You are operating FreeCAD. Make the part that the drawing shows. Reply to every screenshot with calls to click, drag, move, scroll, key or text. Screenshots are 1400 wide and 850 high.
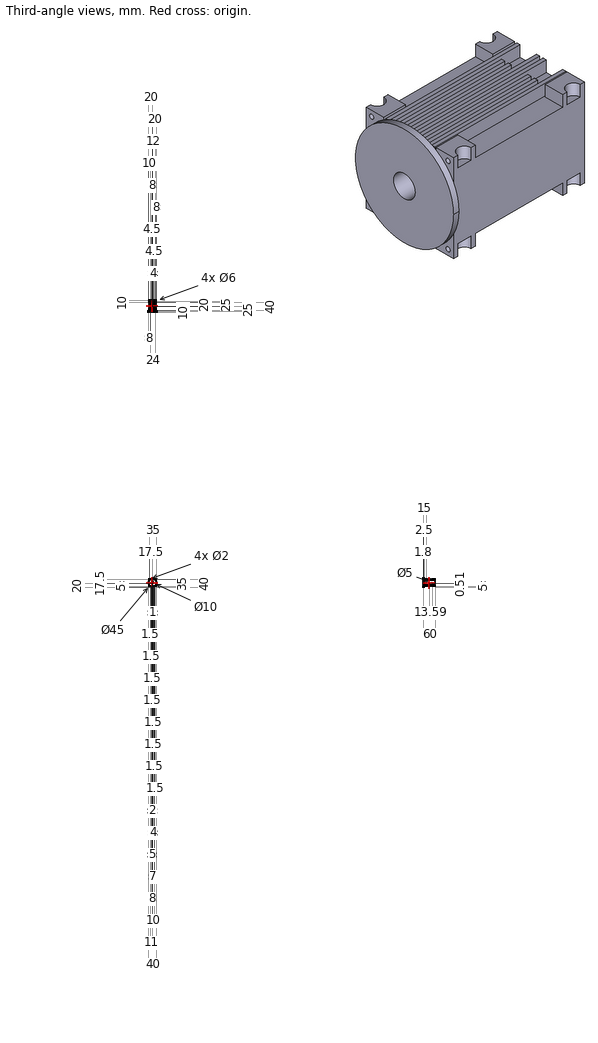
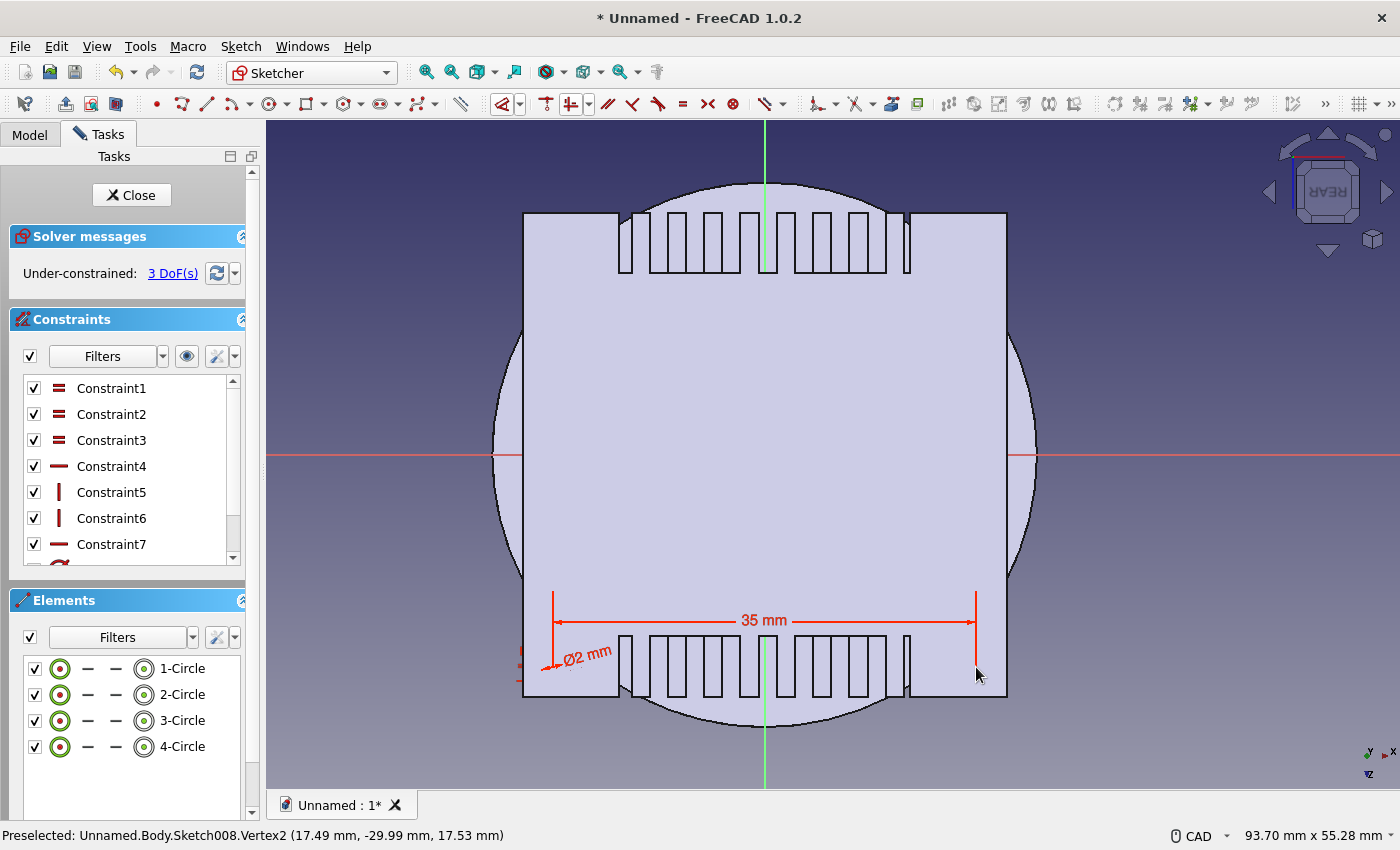
click(976, 667)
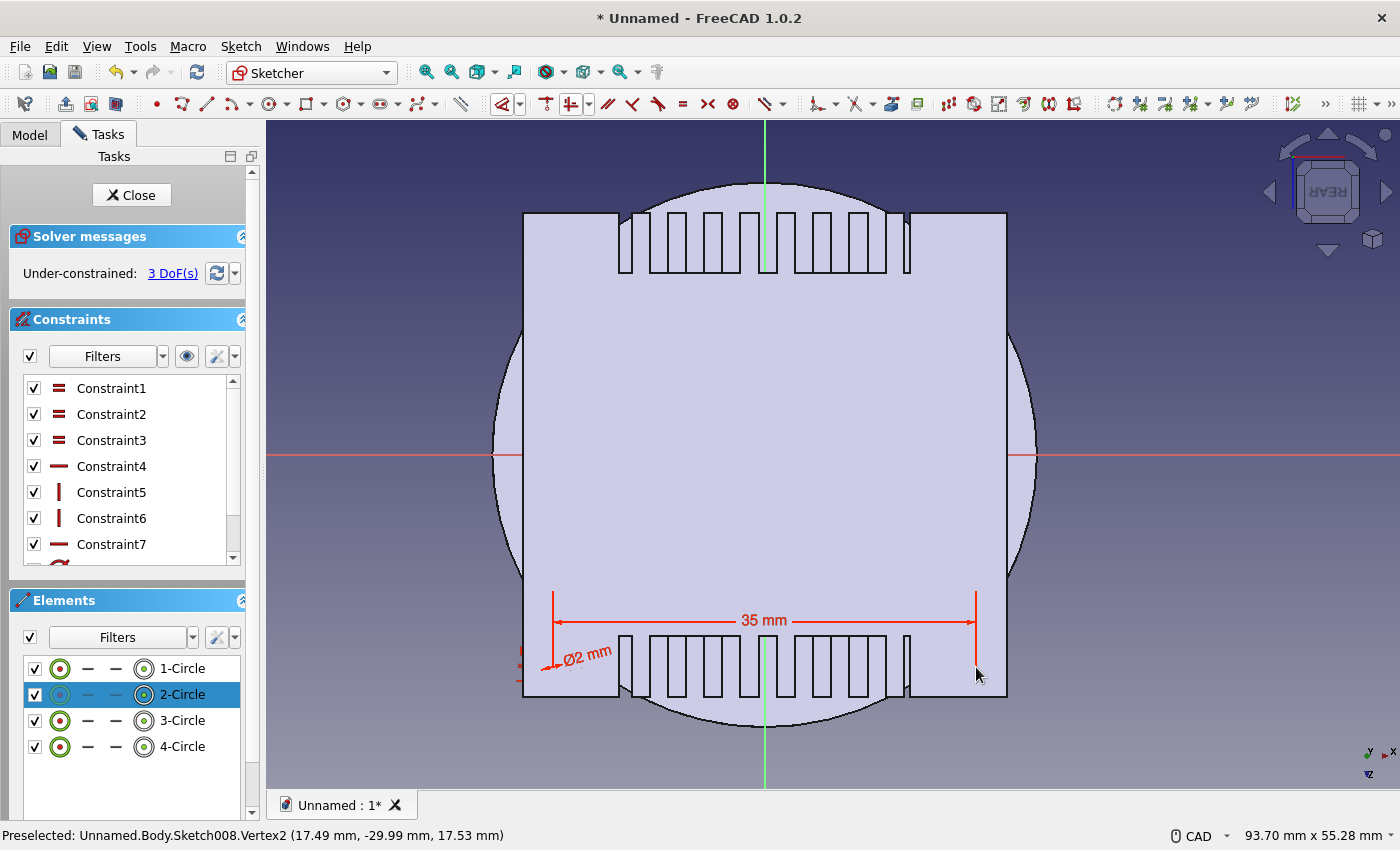
click(976, 244)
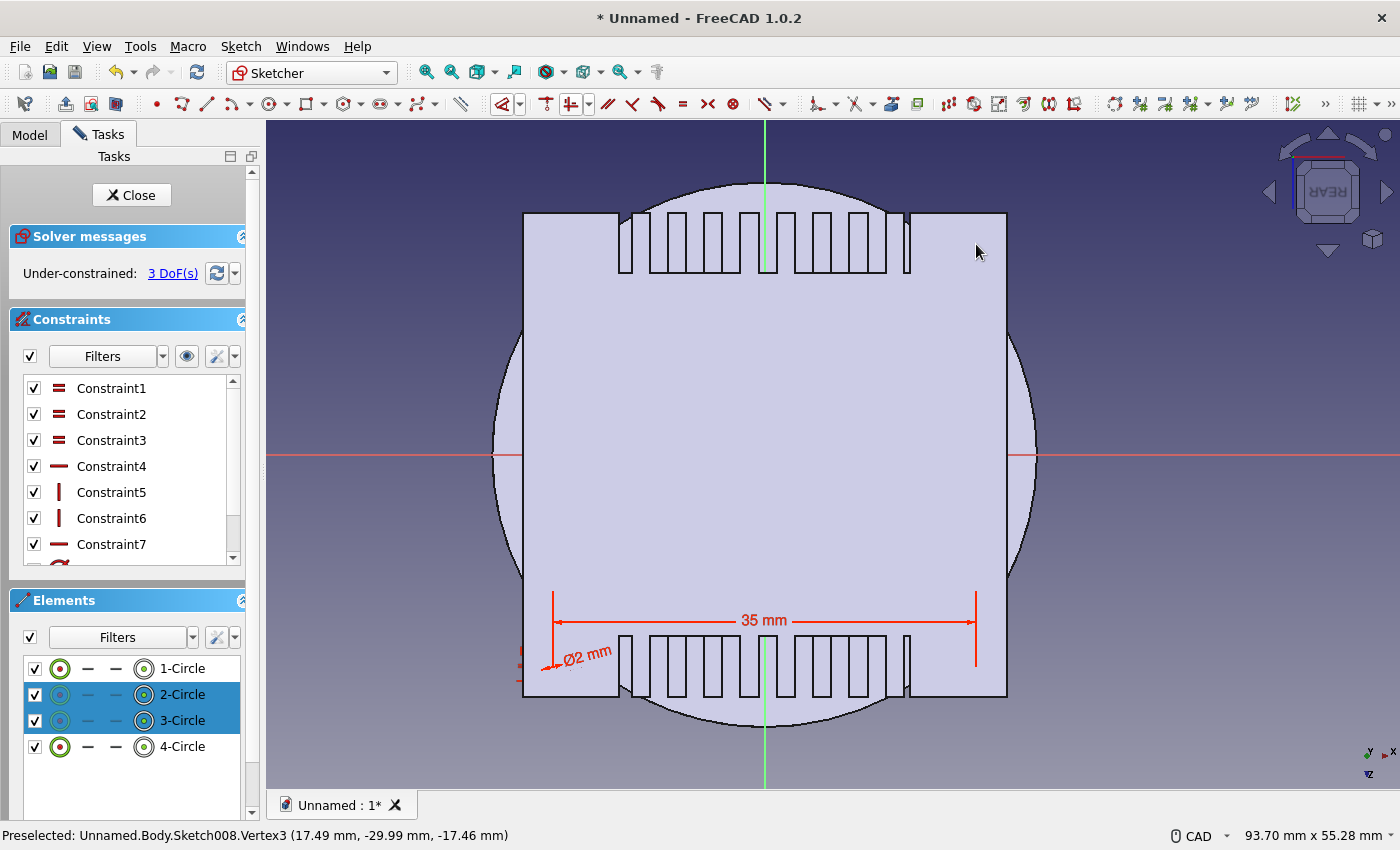
key(i)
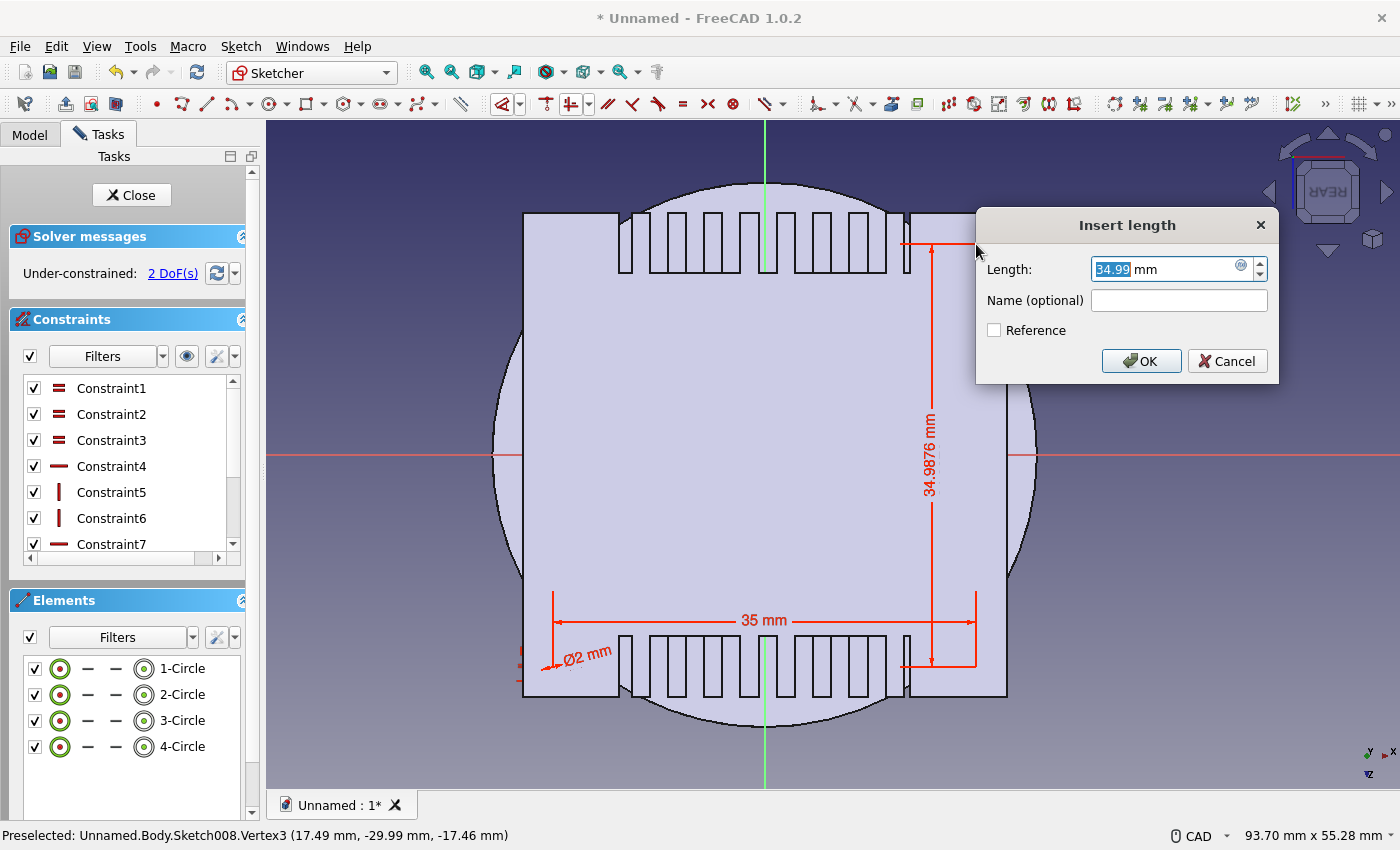
text(35)
key(Return)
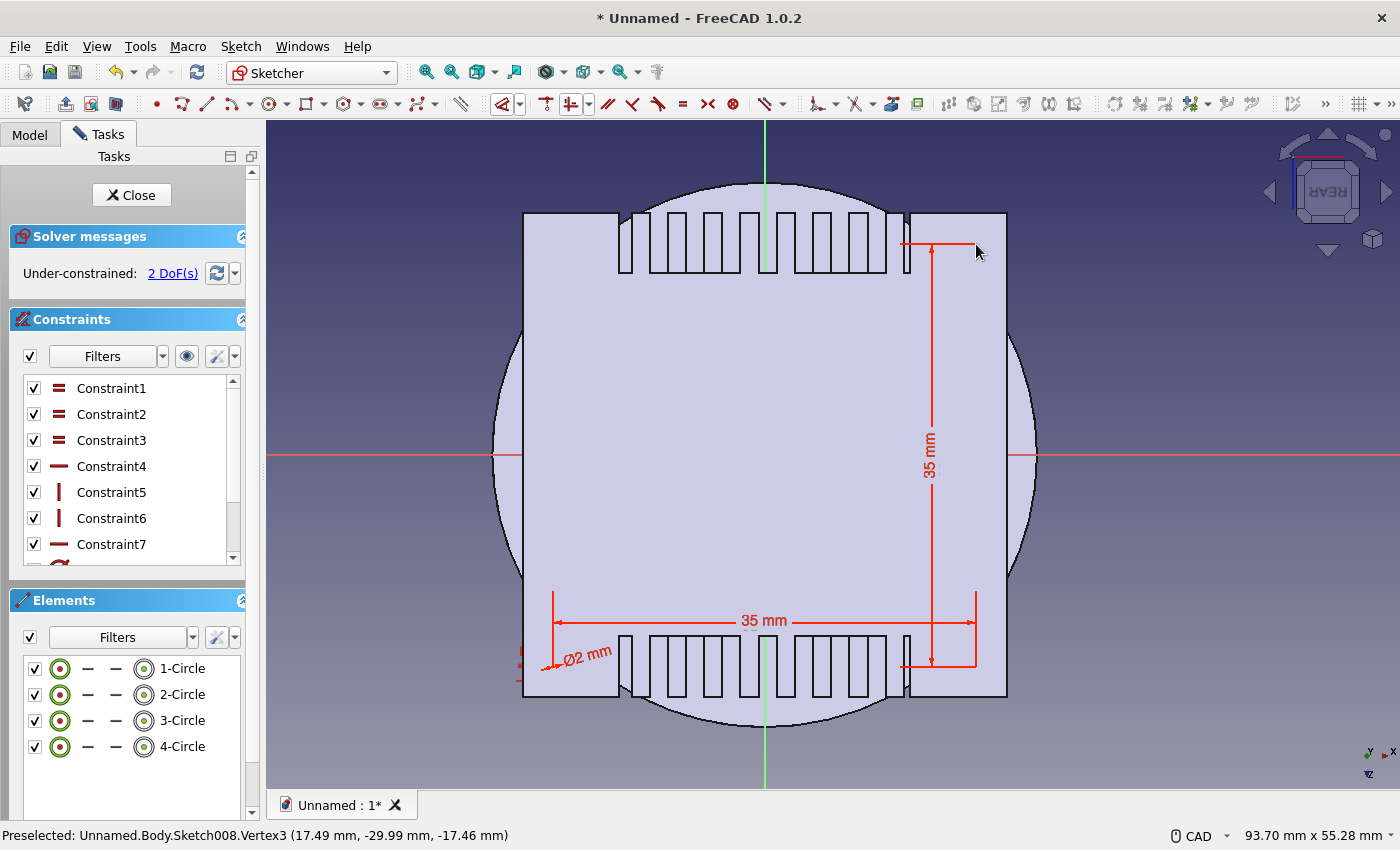
click(553, 667)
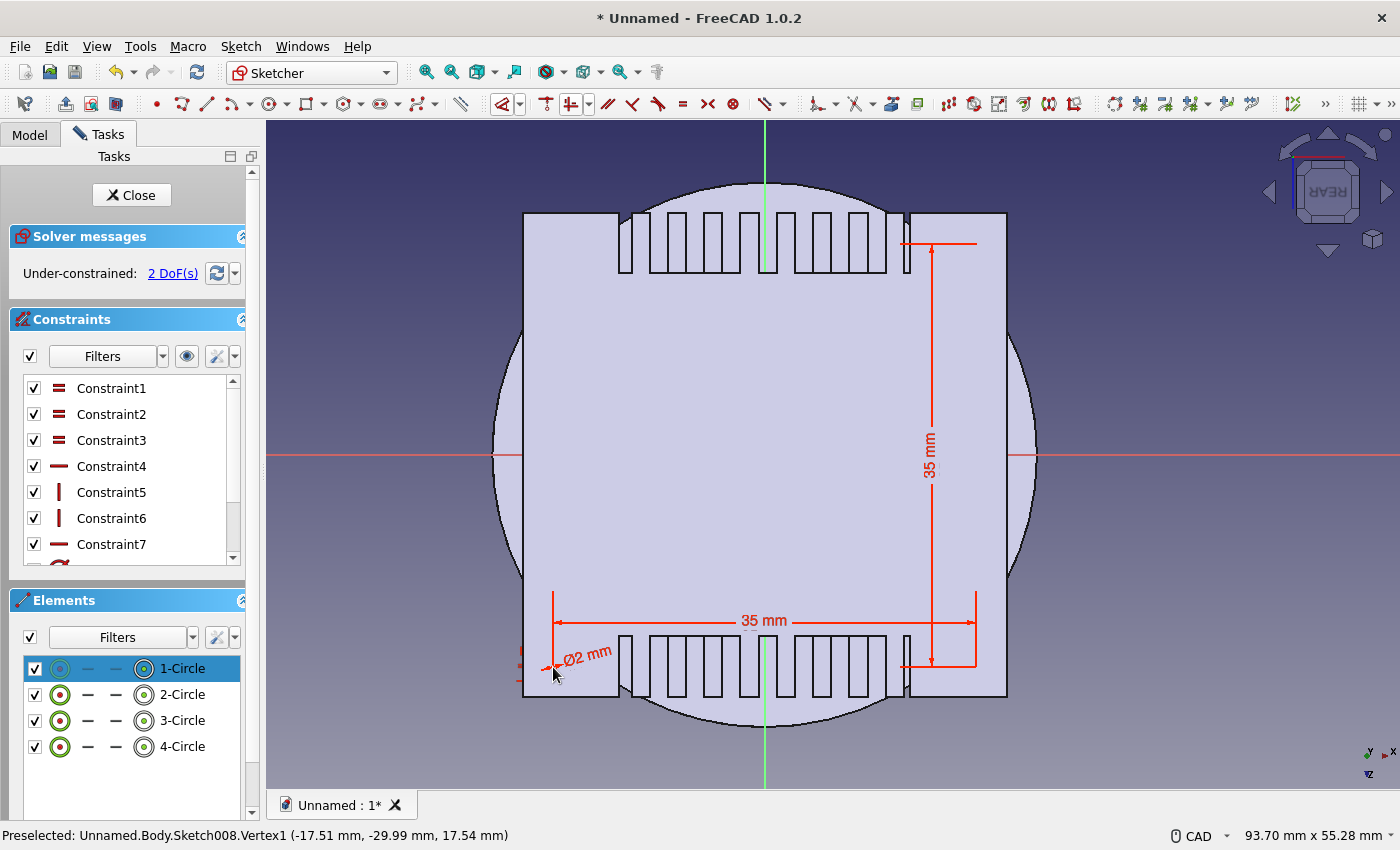
click(520, 104)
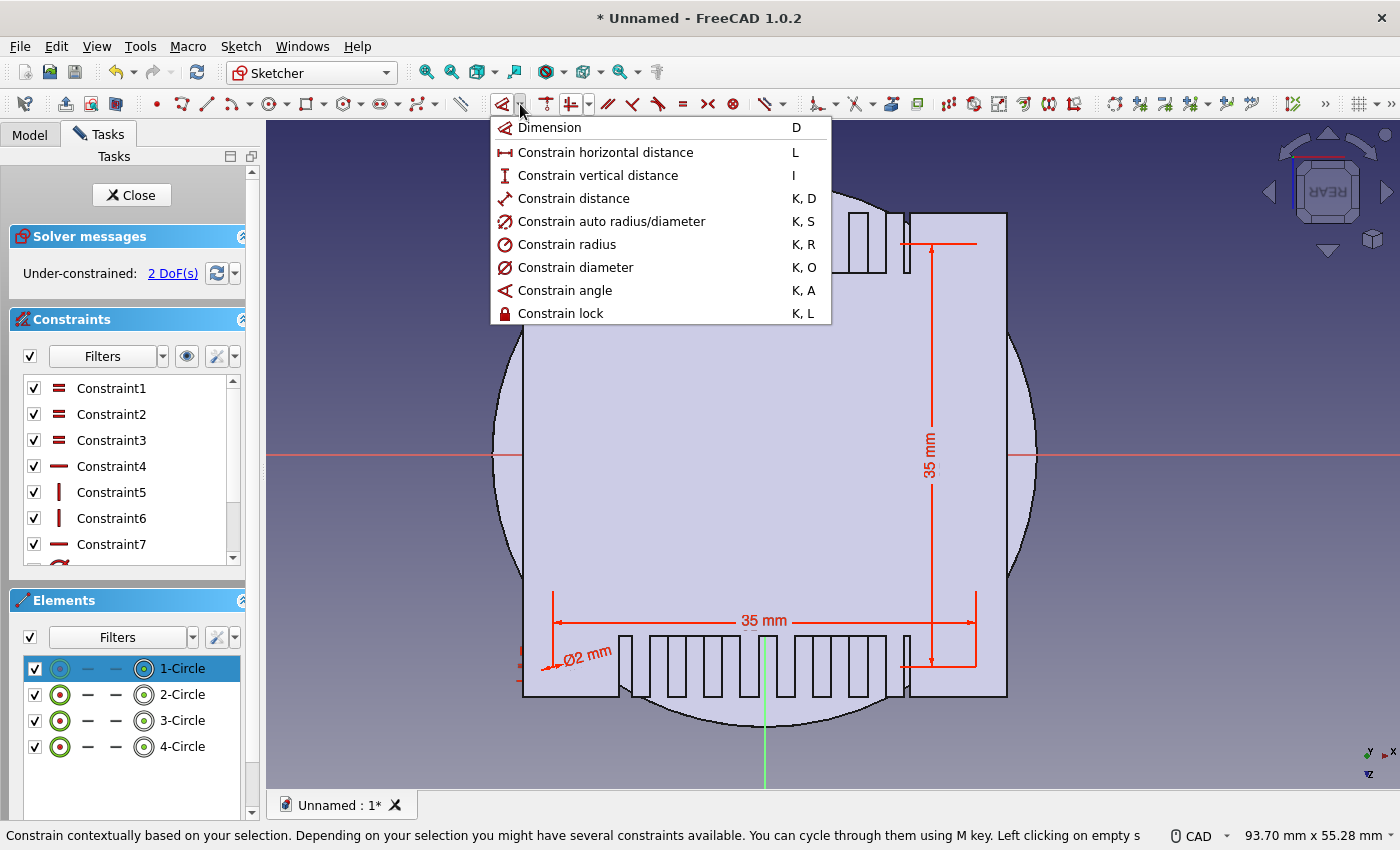
click(661, 152)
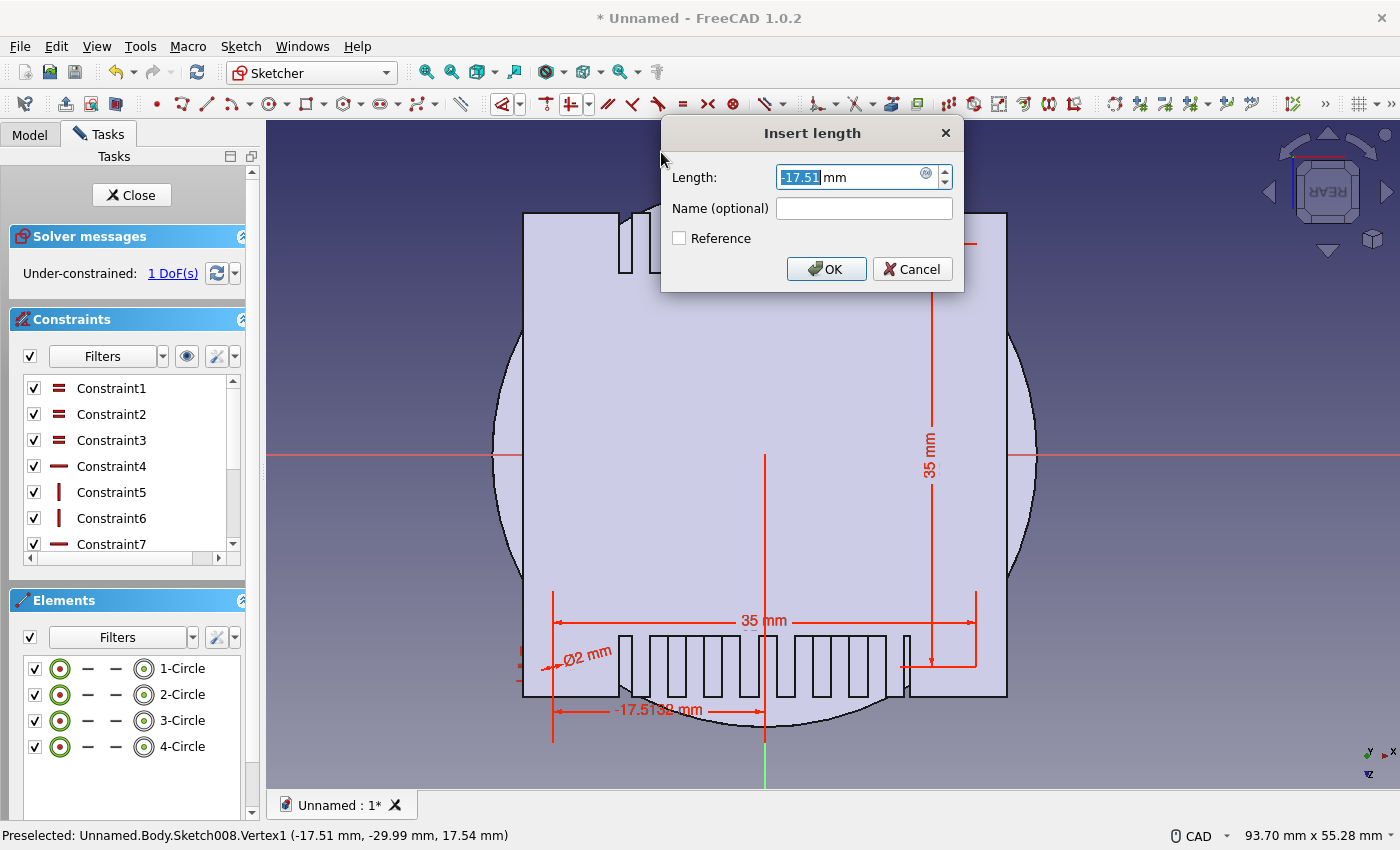
text(-17.5)
key(Return)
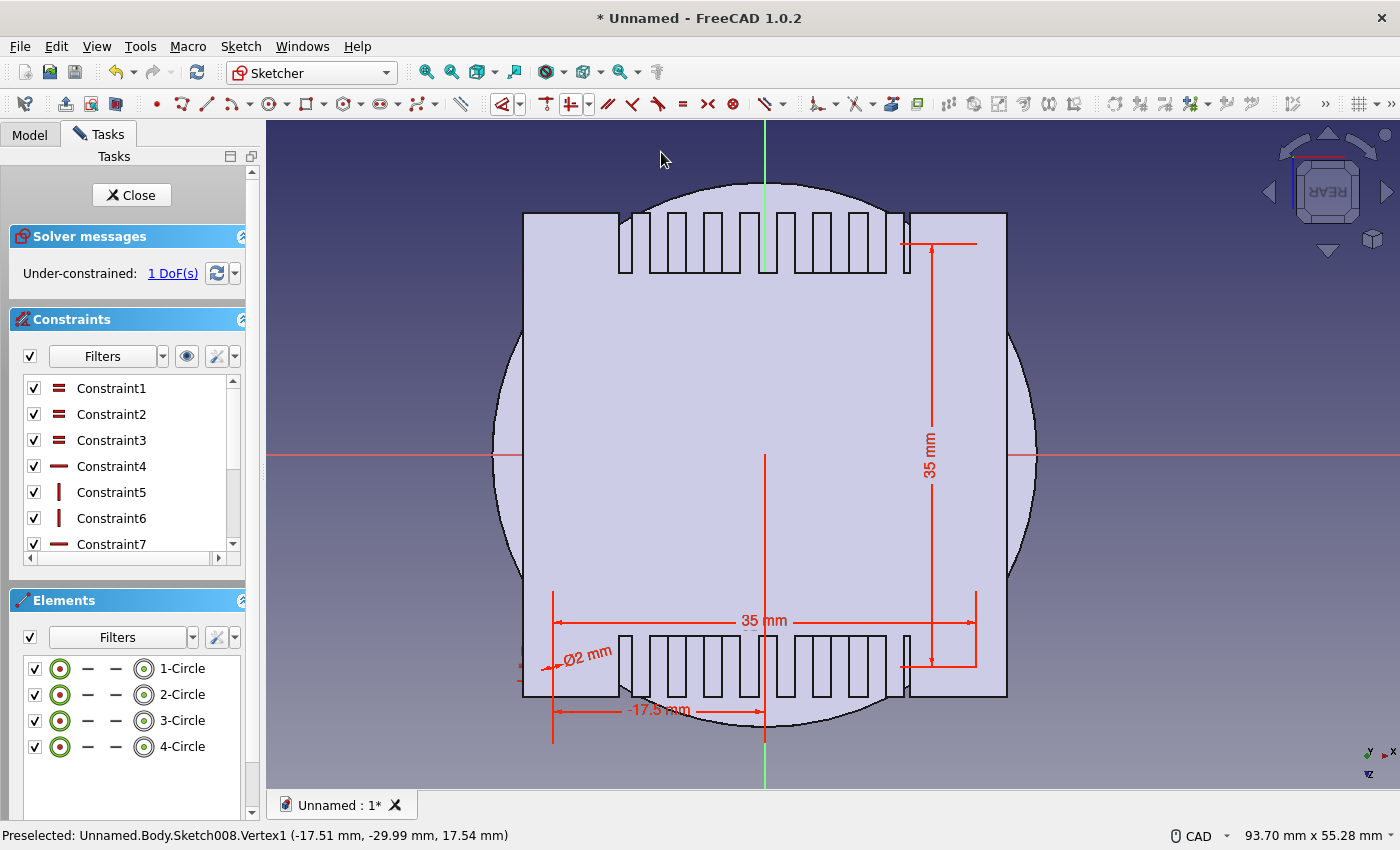
click(553, 667)